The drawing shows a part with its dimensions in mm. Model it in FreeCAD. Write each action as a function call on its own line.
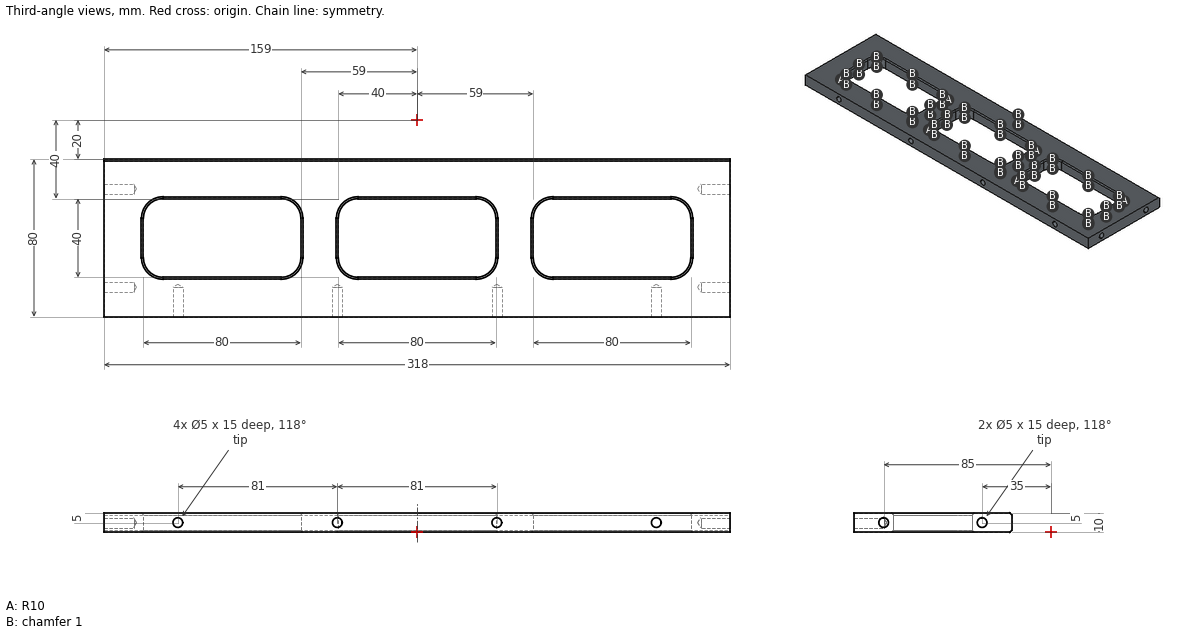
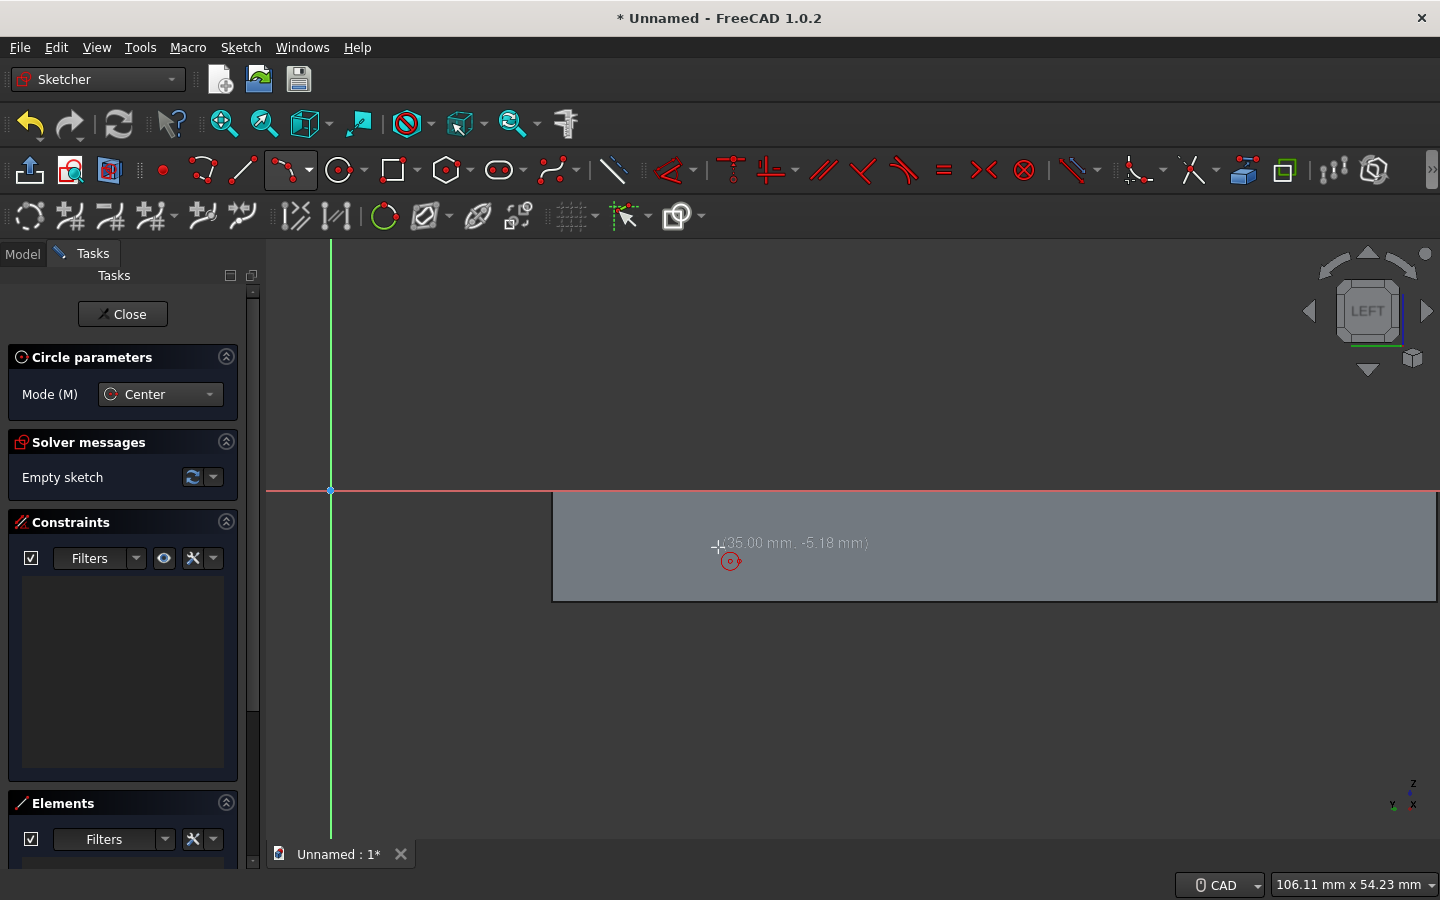
click(718, 546)
click(737, 527)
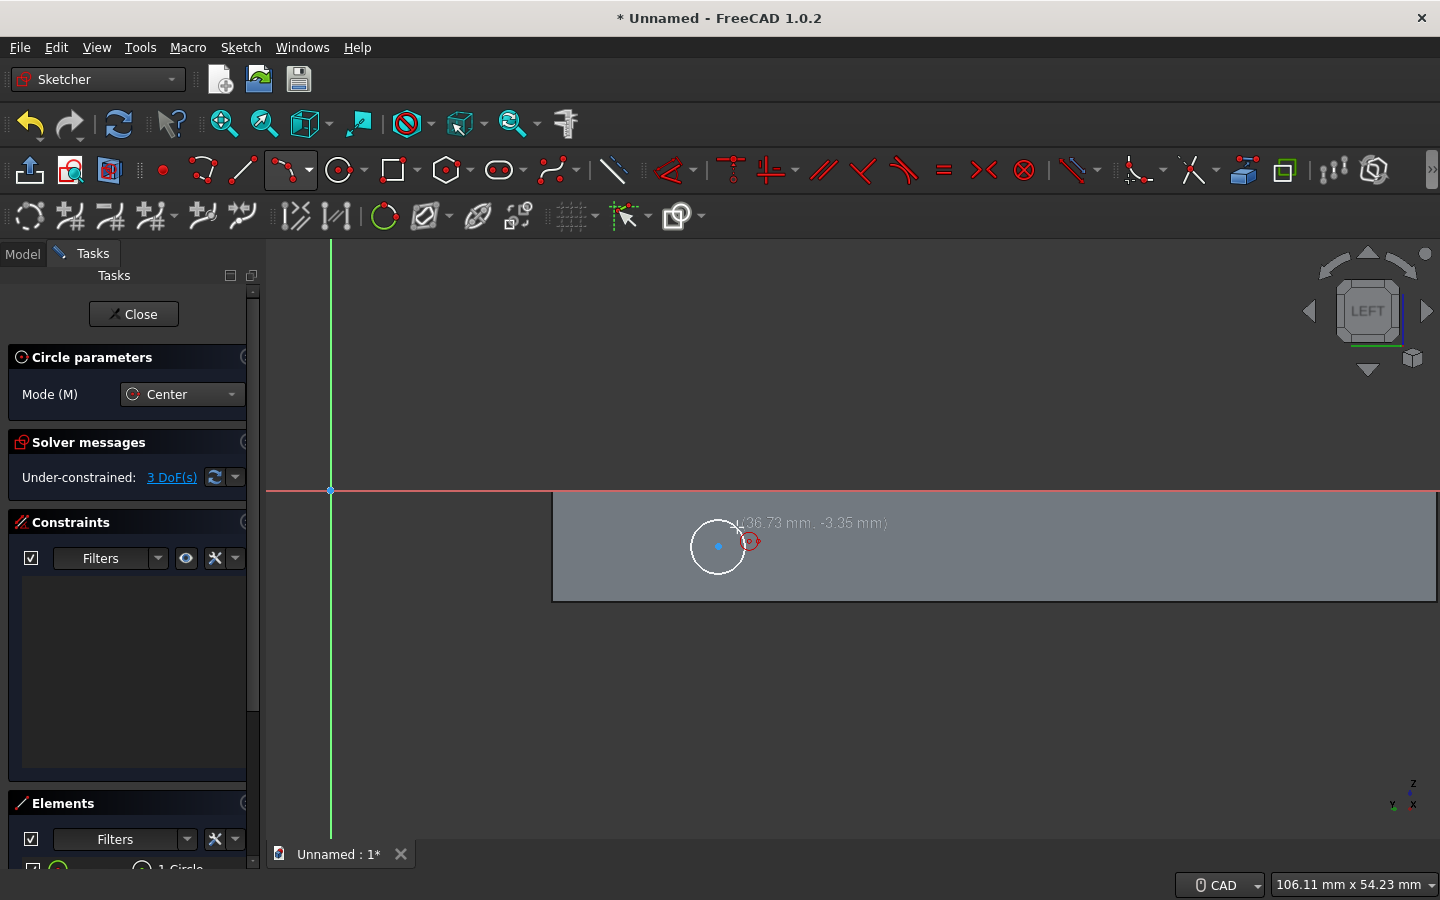
click(1271, 546)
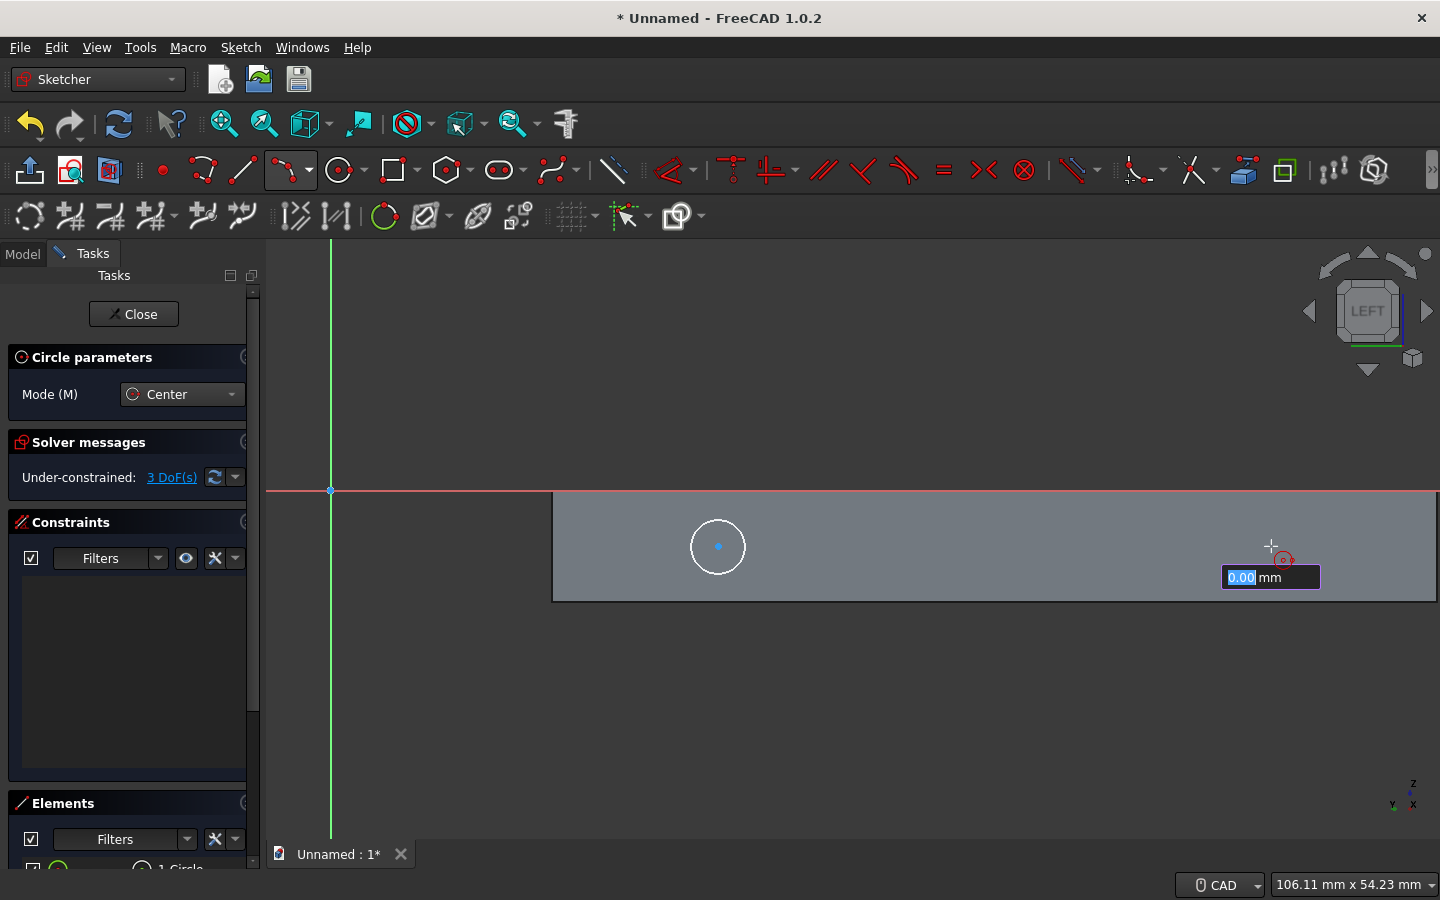
scroll(723, 552, down, 2)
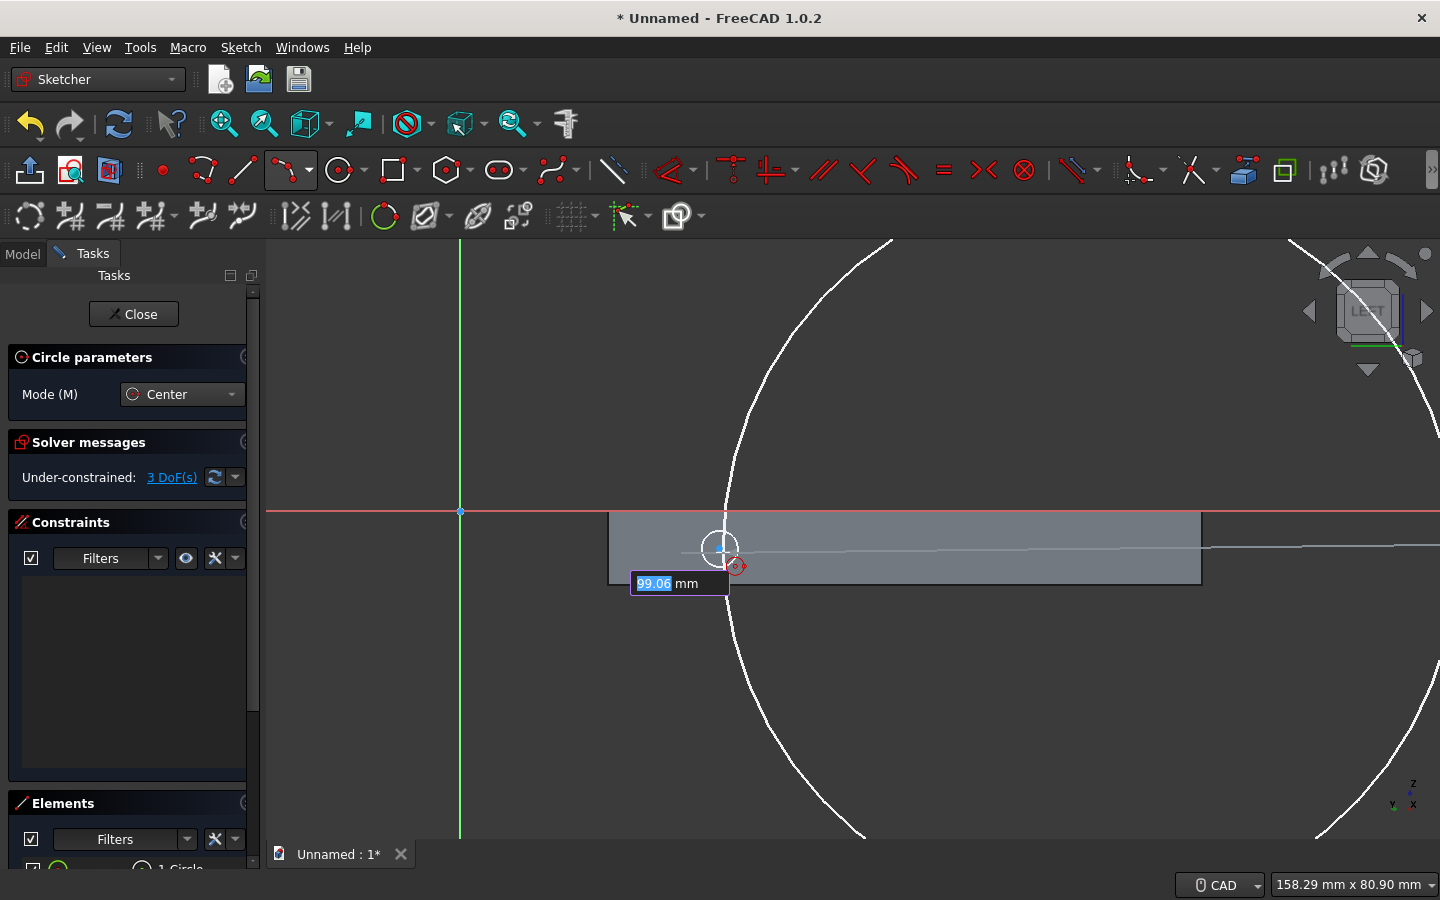
click(1104, 535)
key(Escape)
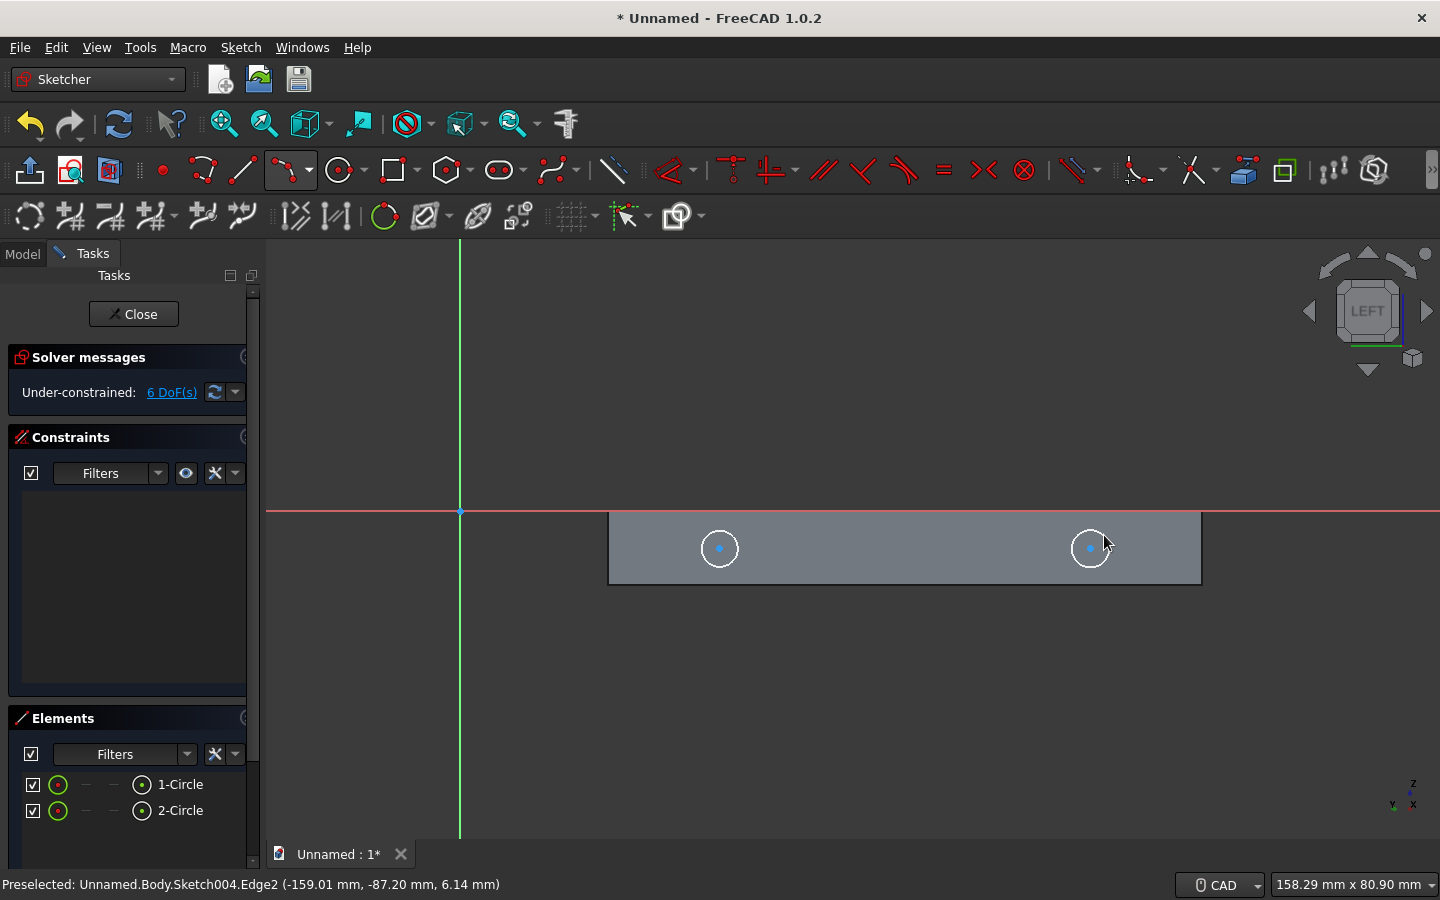
click(732, 536)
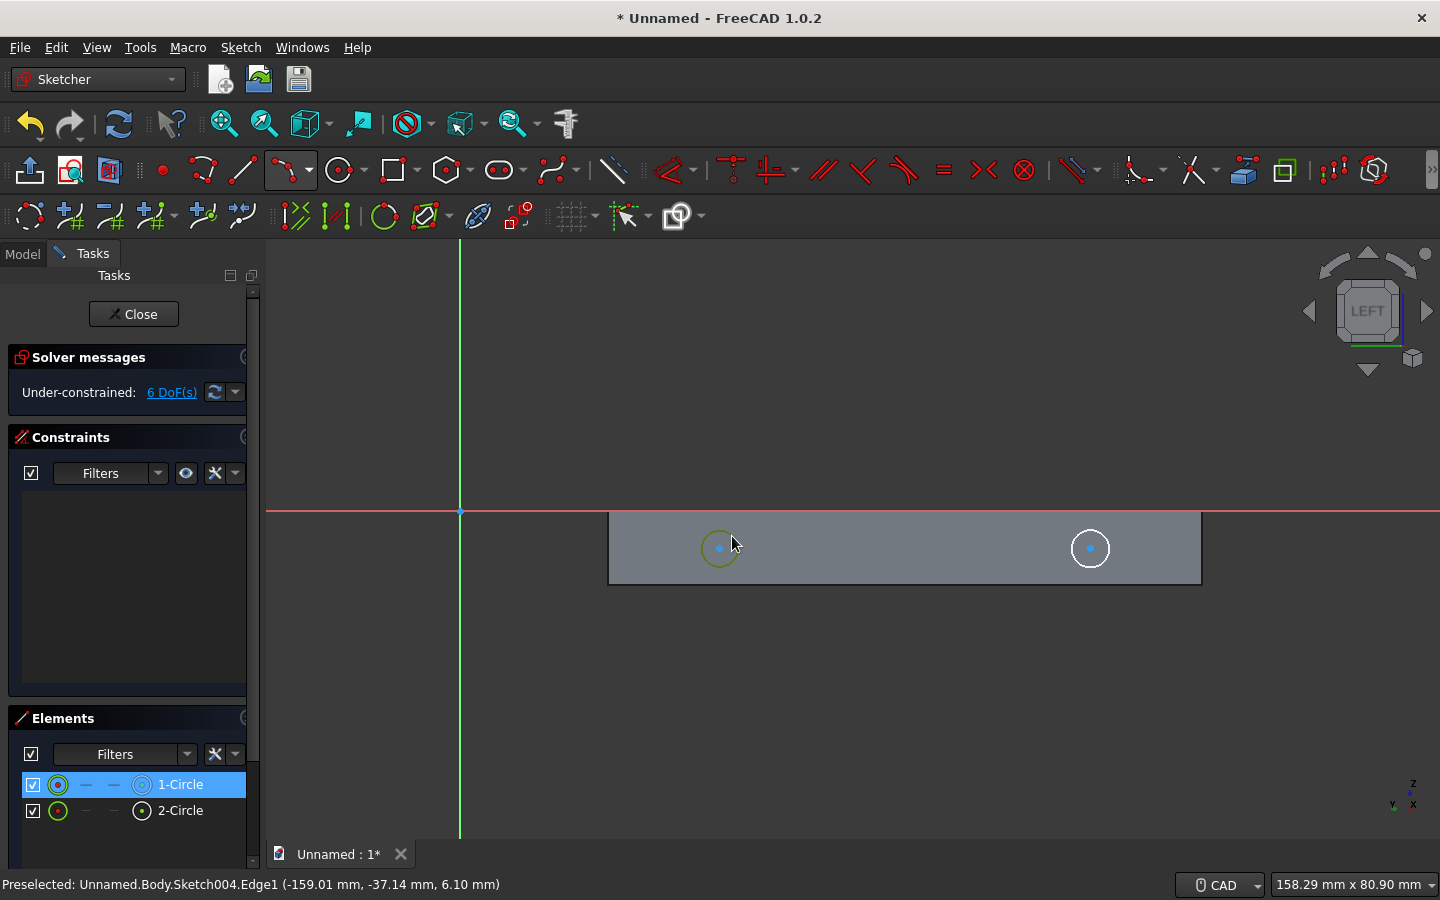
click(1104, 536)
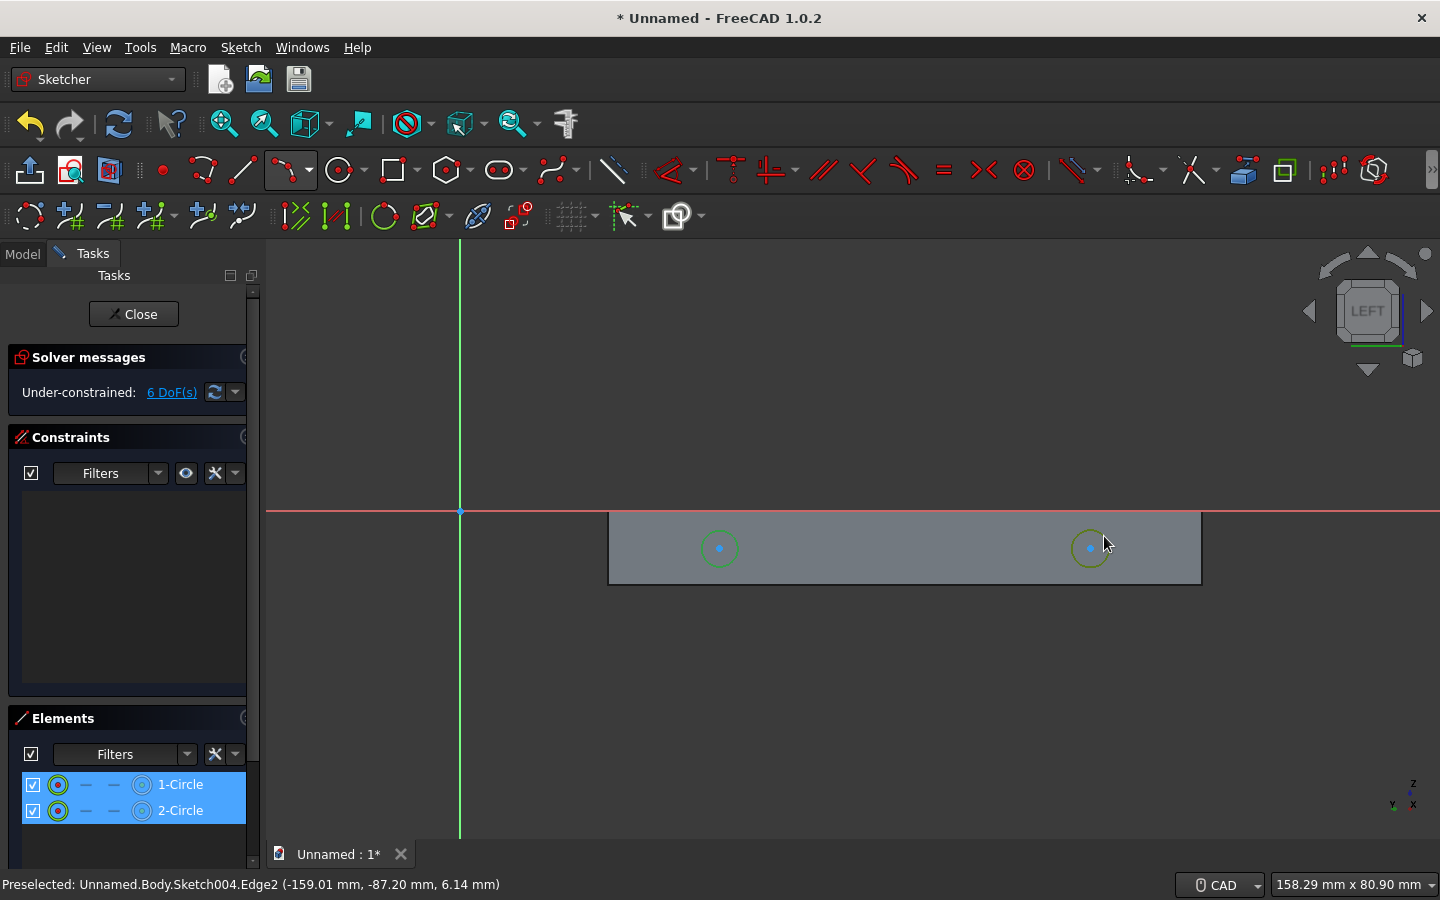
key(e)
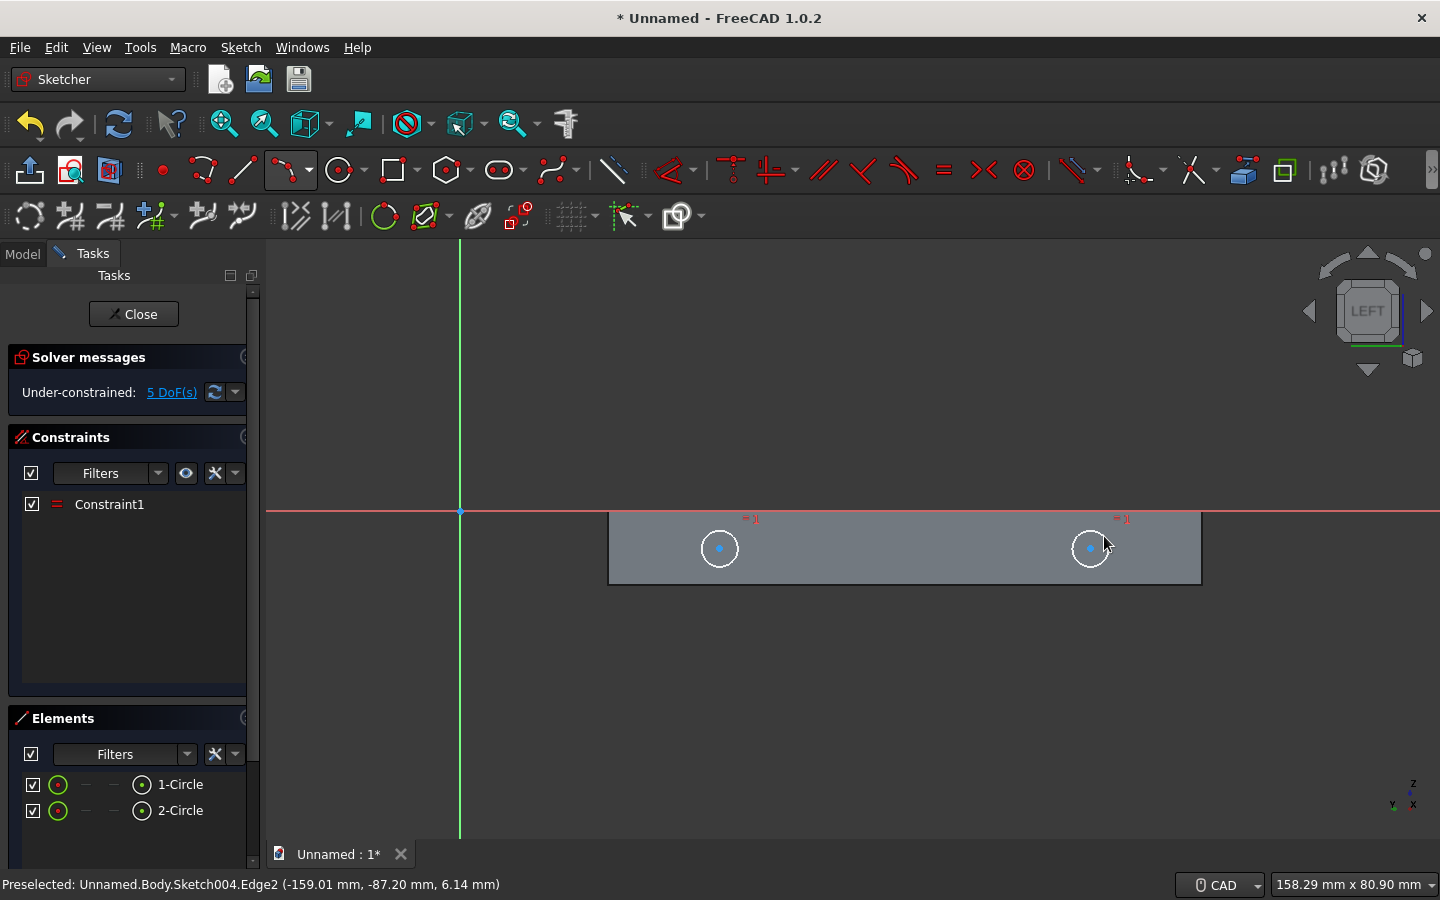
click(668, 170)